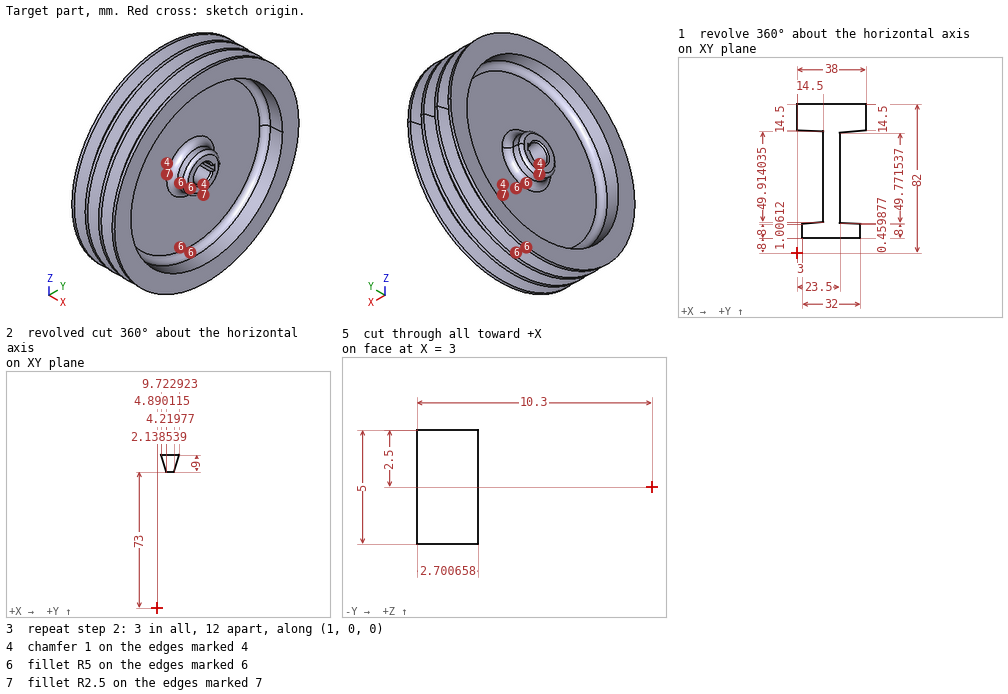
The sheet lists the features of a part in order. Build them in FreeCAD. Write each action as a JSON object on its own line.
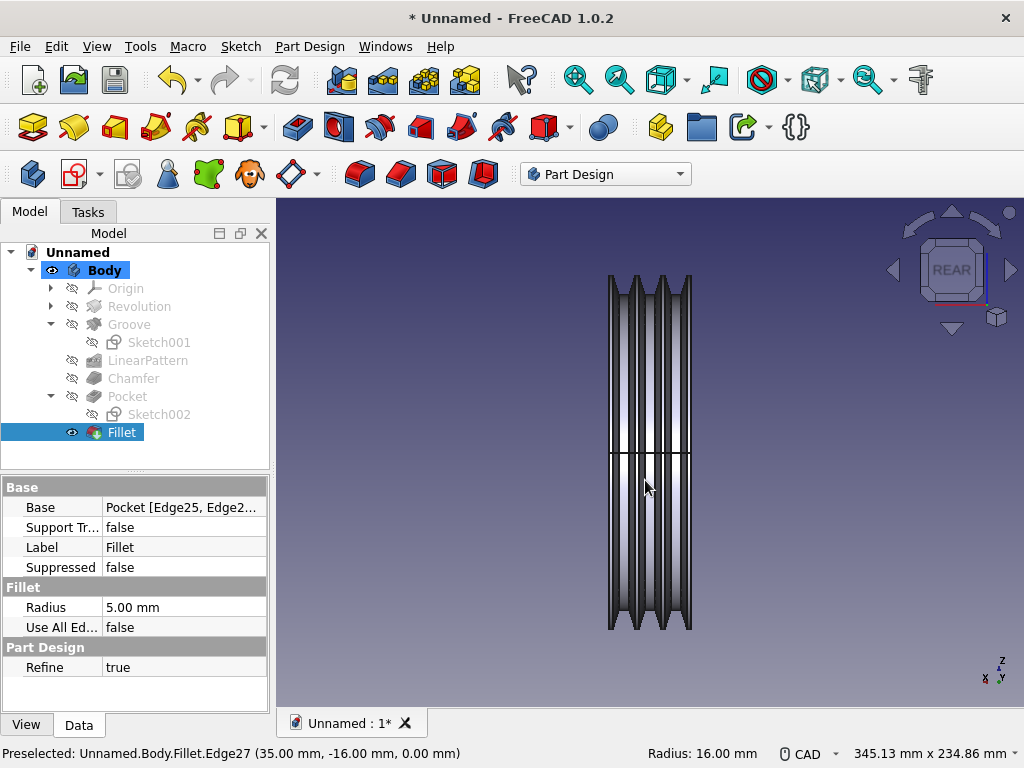
{"action": "key", "text": "6"}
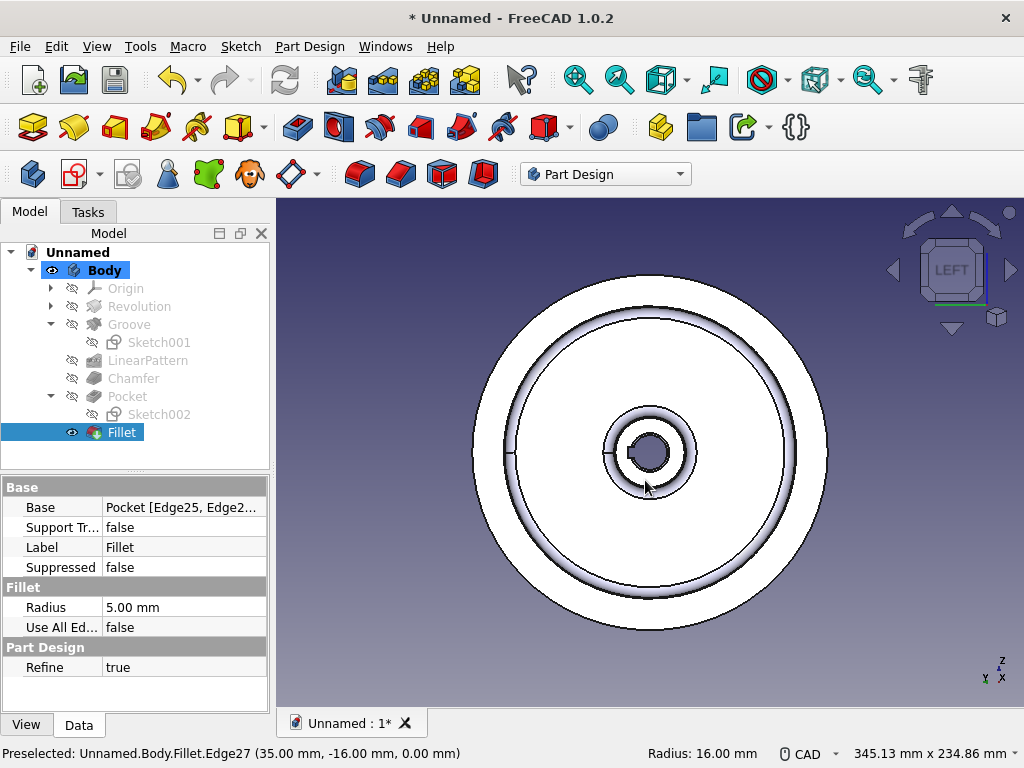
{"action": "left_click", "coordinate": [685, 451], "text": "ctrl"}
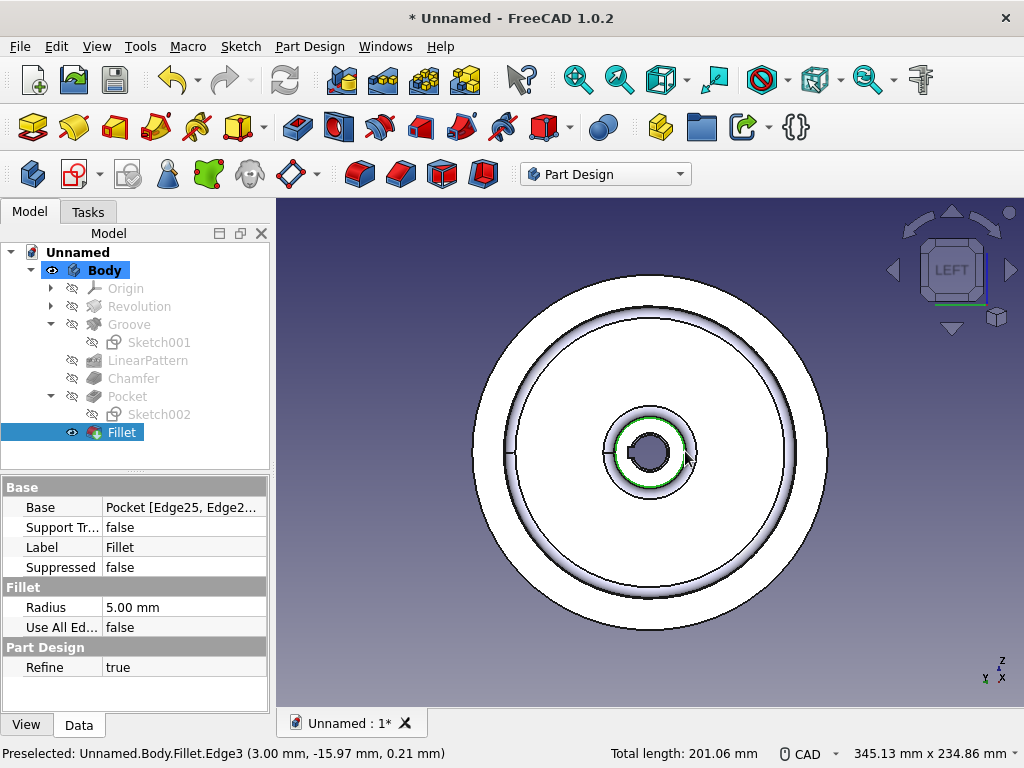
{"action": "left_click", "coordinate": [360, 174]}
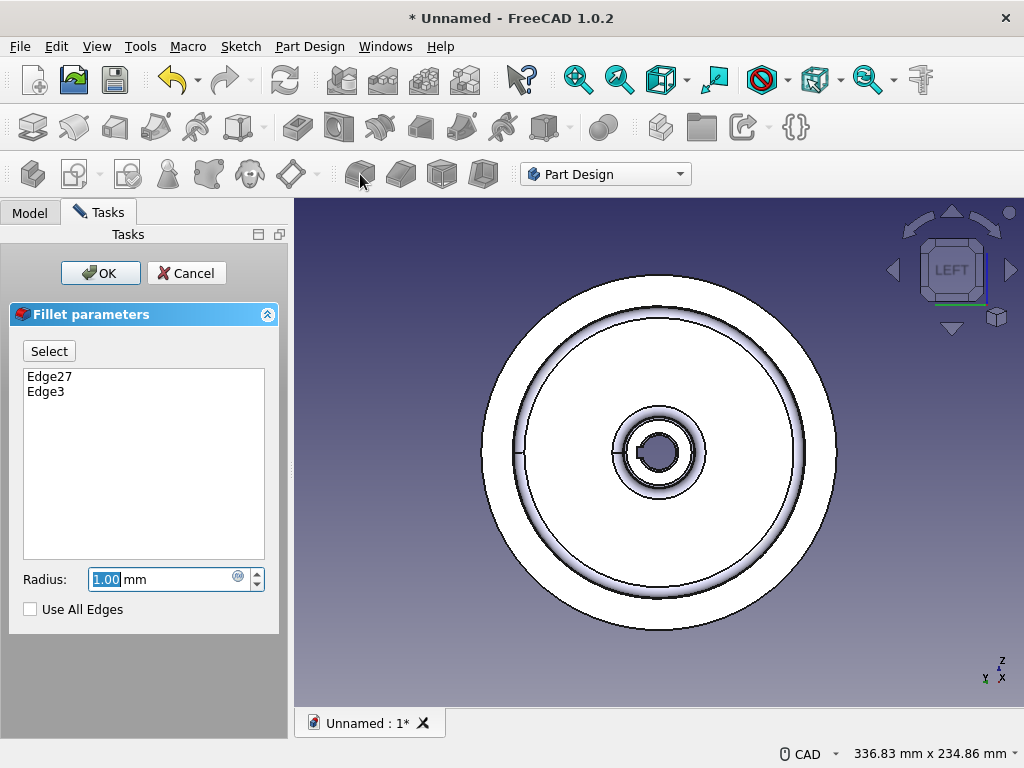
{"action": "type", "text": "2.5"}
{"action": "key", "text": "Tab"}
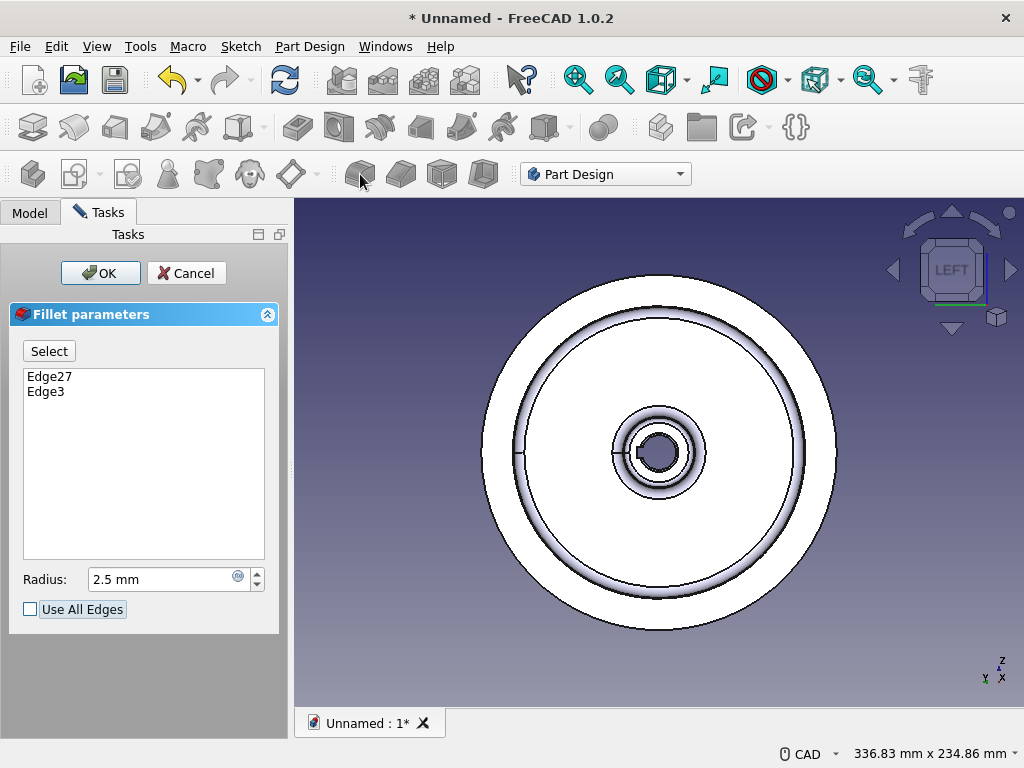
{"action": "left_click", "coordinate": [101, 273]}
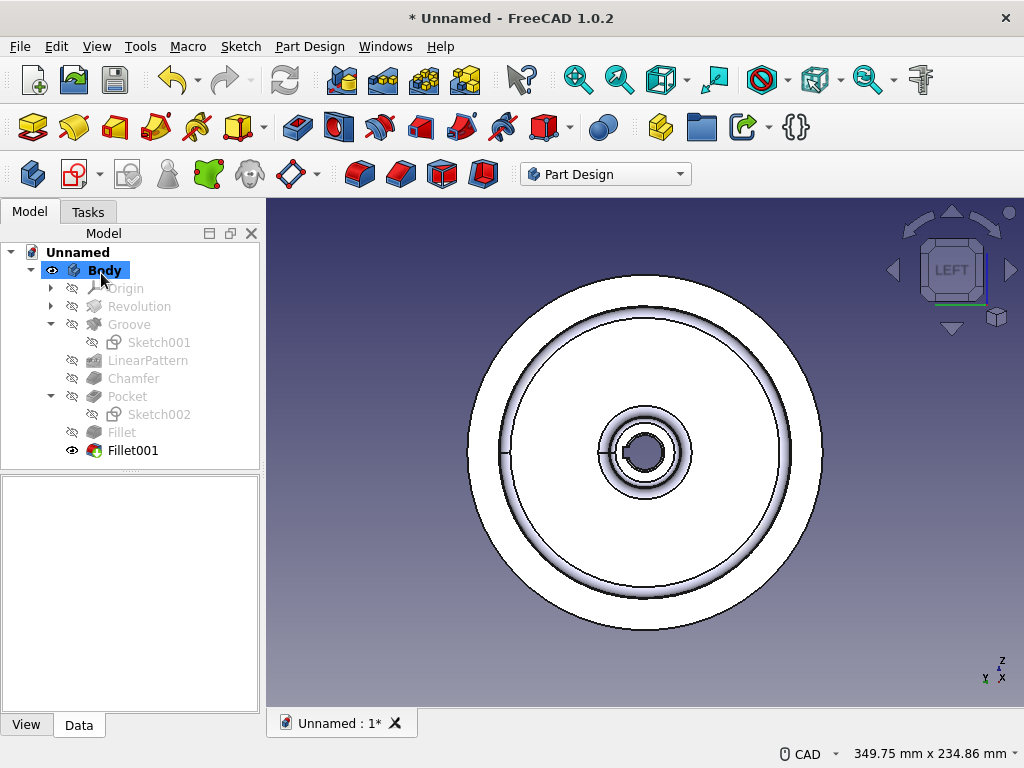
{"action": "key", "text": "0"}